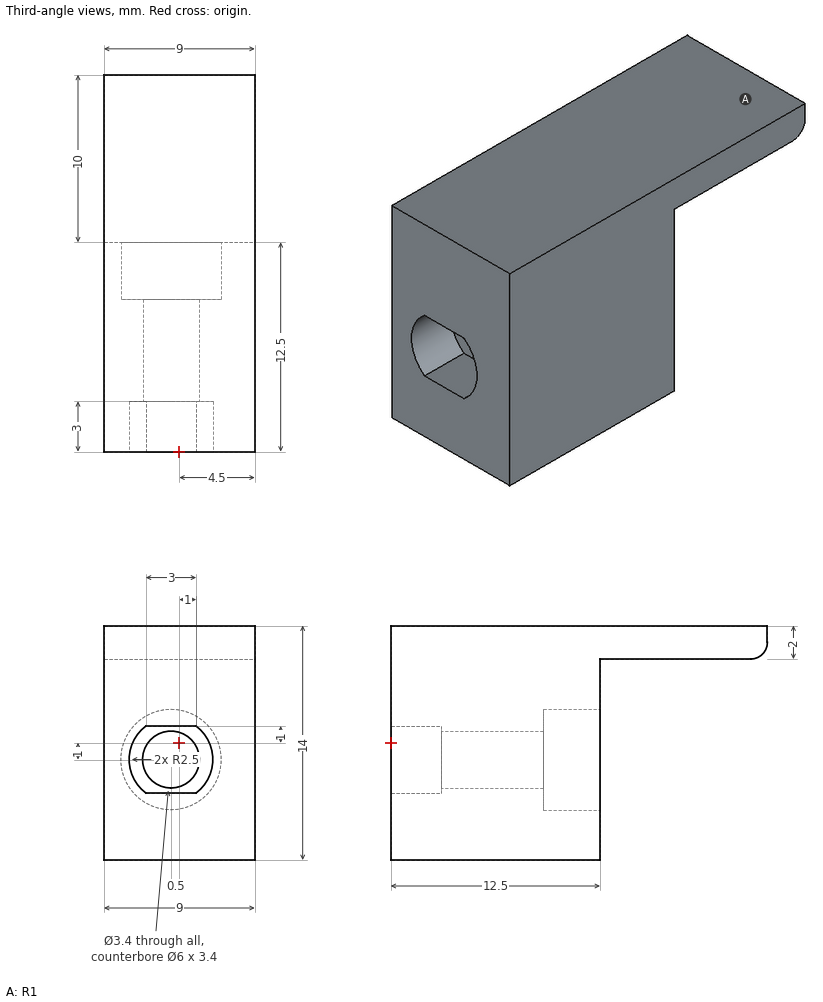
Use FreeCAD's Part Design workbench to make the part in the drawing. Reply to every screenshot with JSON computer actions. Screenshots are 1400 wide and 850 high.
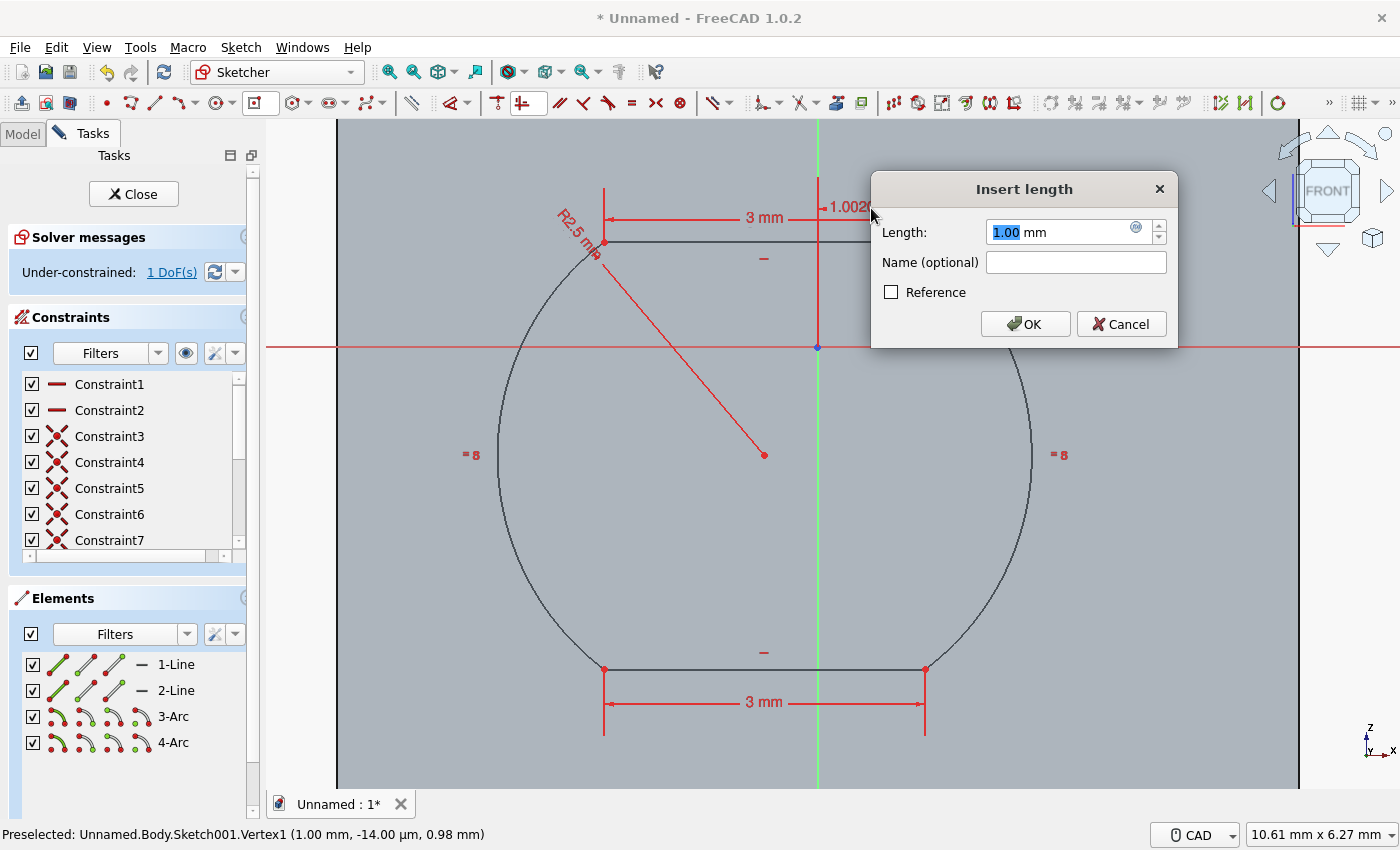
{"action": "type", "text": "1"}
{"action": "key", "text": "Return"}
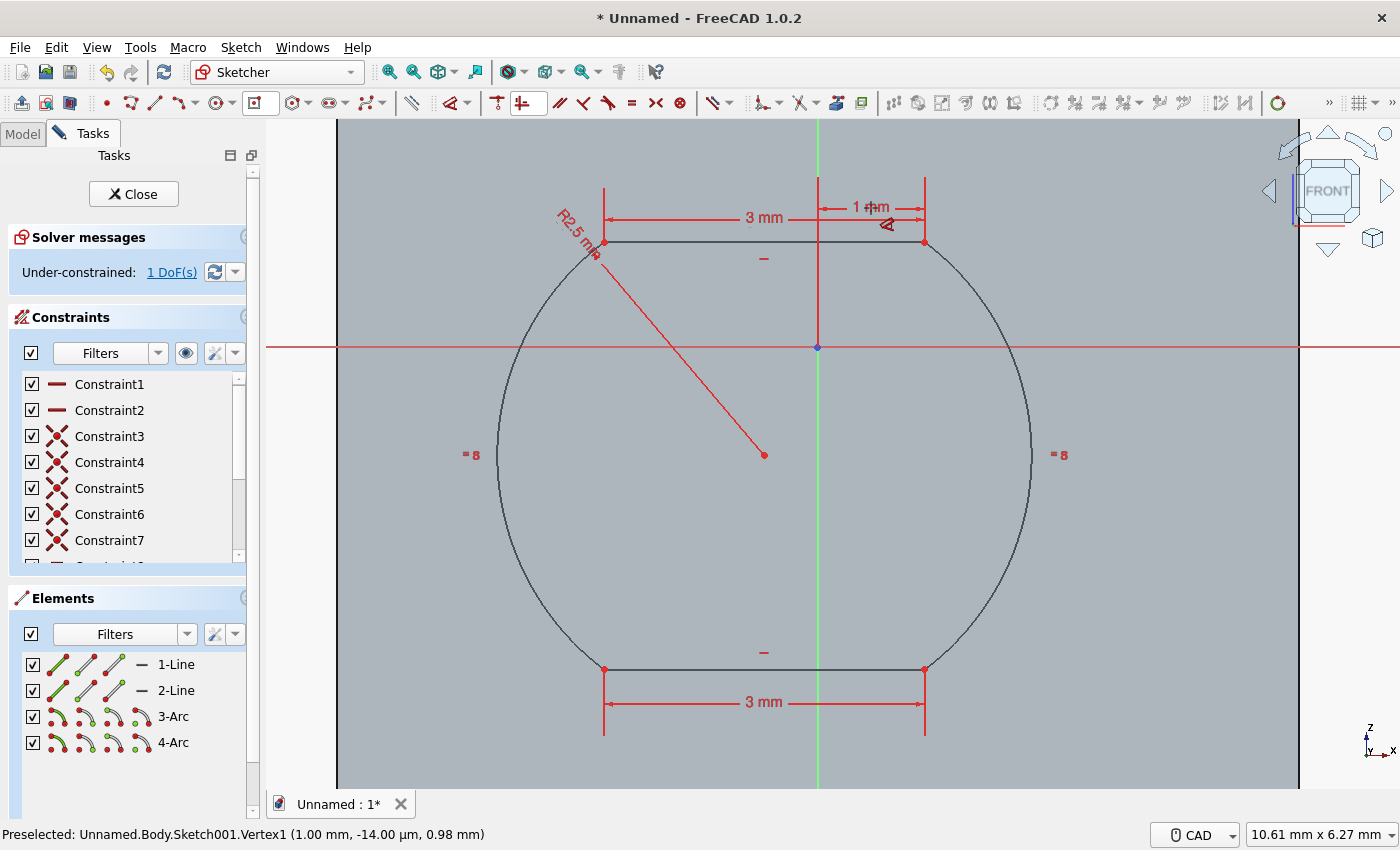
{"action": "left_click", "coordinate": [925, 242]}
{"action": "left_click", "coordinate": [959, 295]}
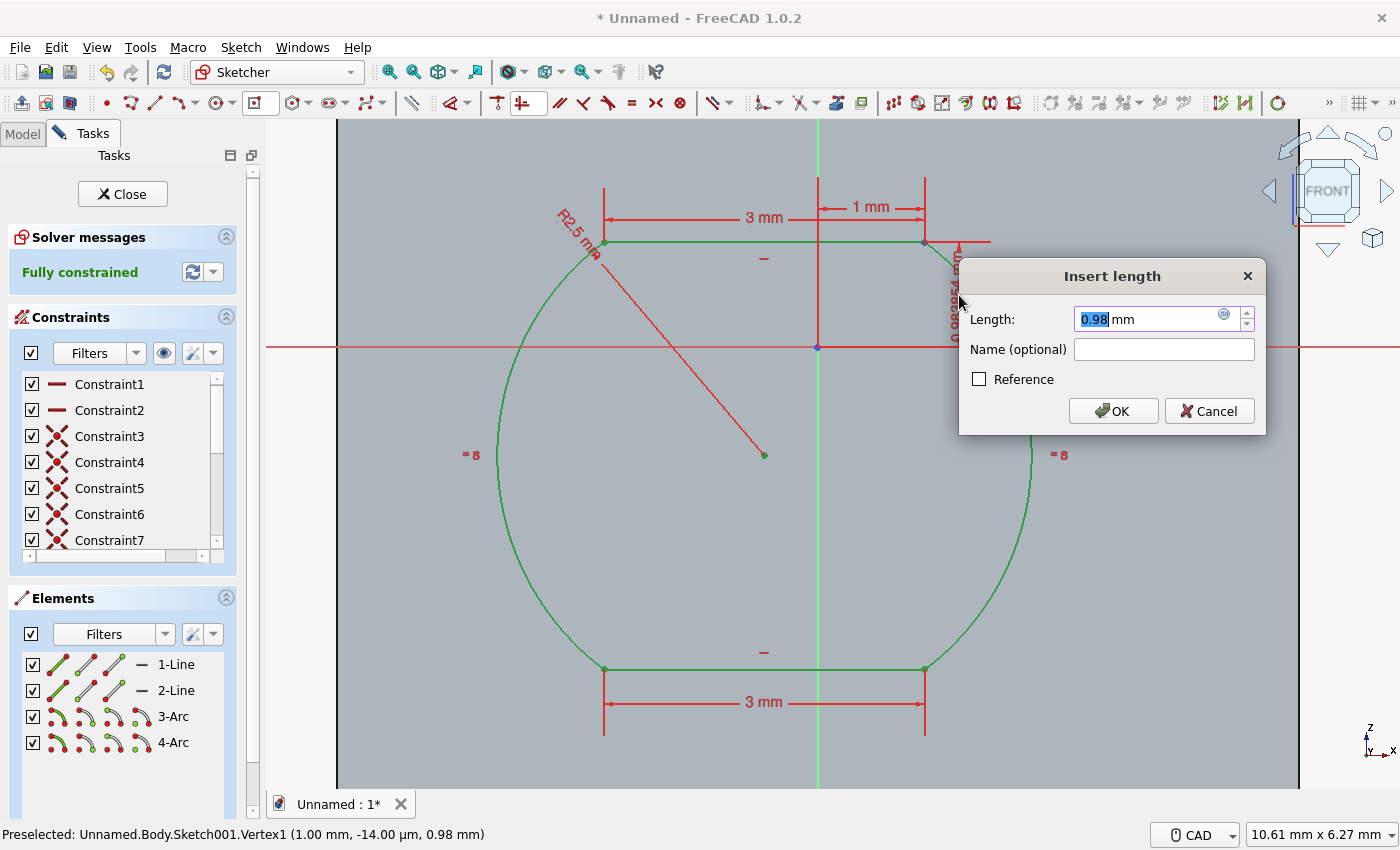
{"action": "type", "text": "1"}
{"action": "key", "text": "Return"}
{"action": "key", "text": "Escape"}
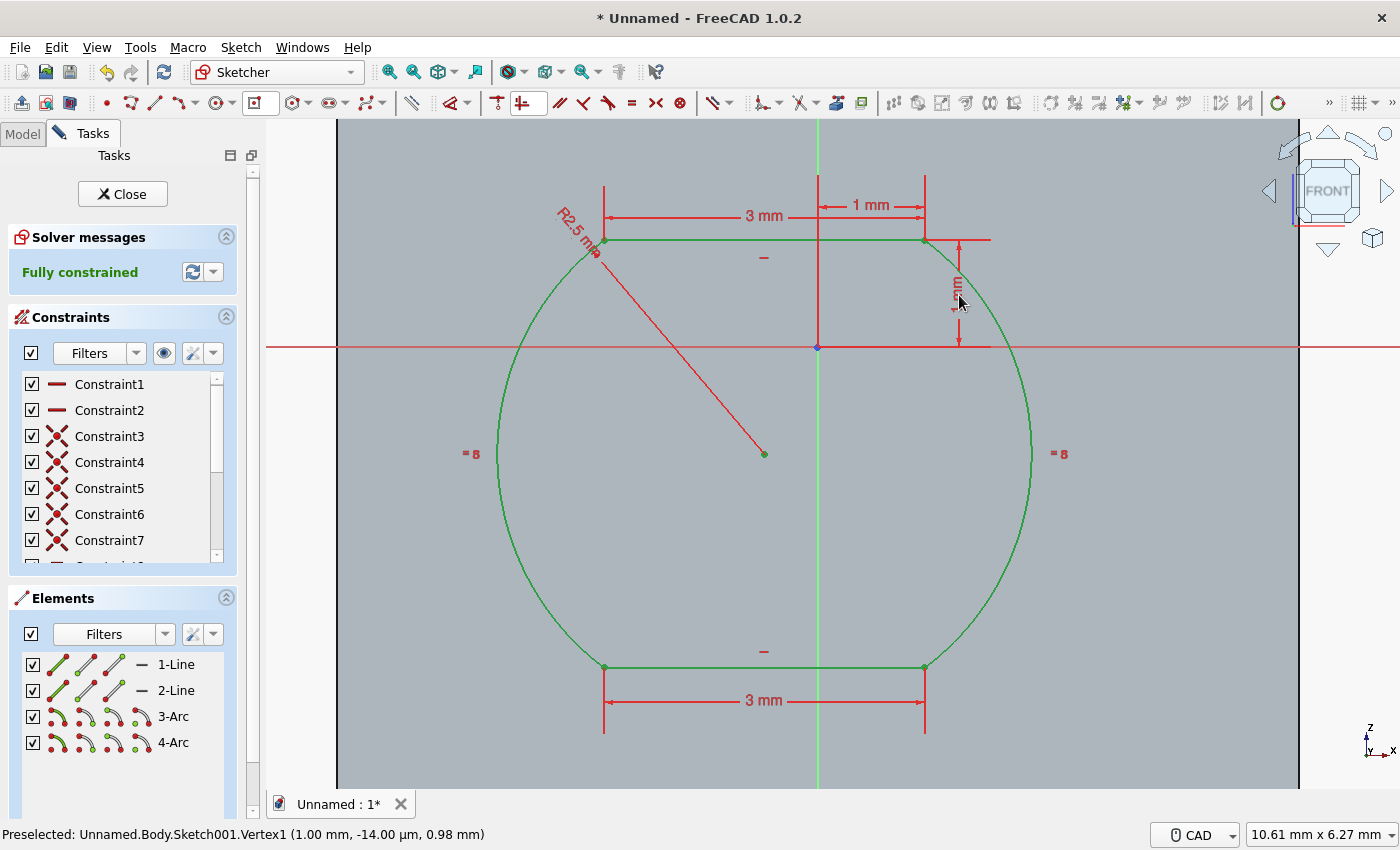
{"action": "left_click", "coordinate": [123, 194]}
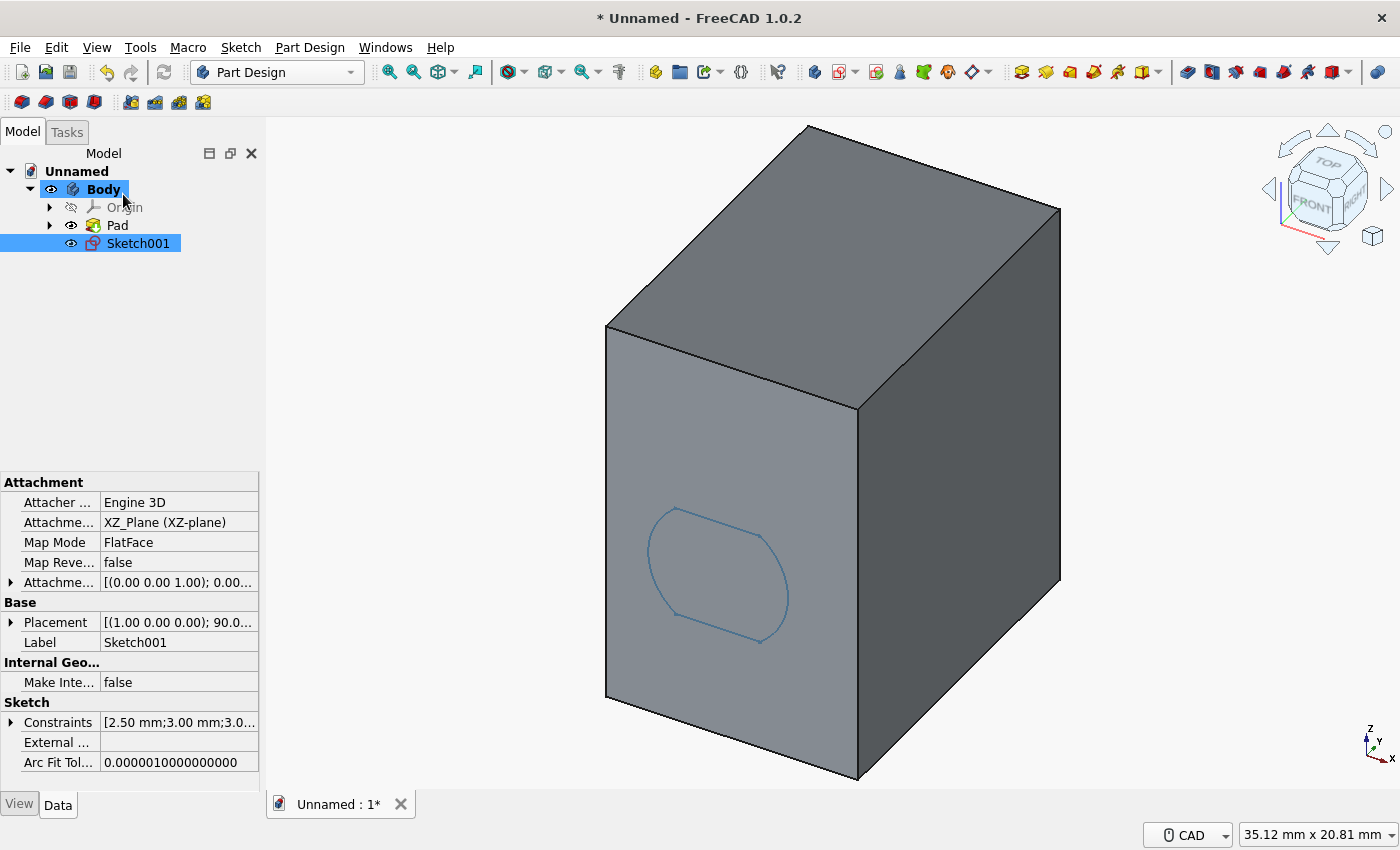
{"action": "left_click", "coordinate": [1188, 72]}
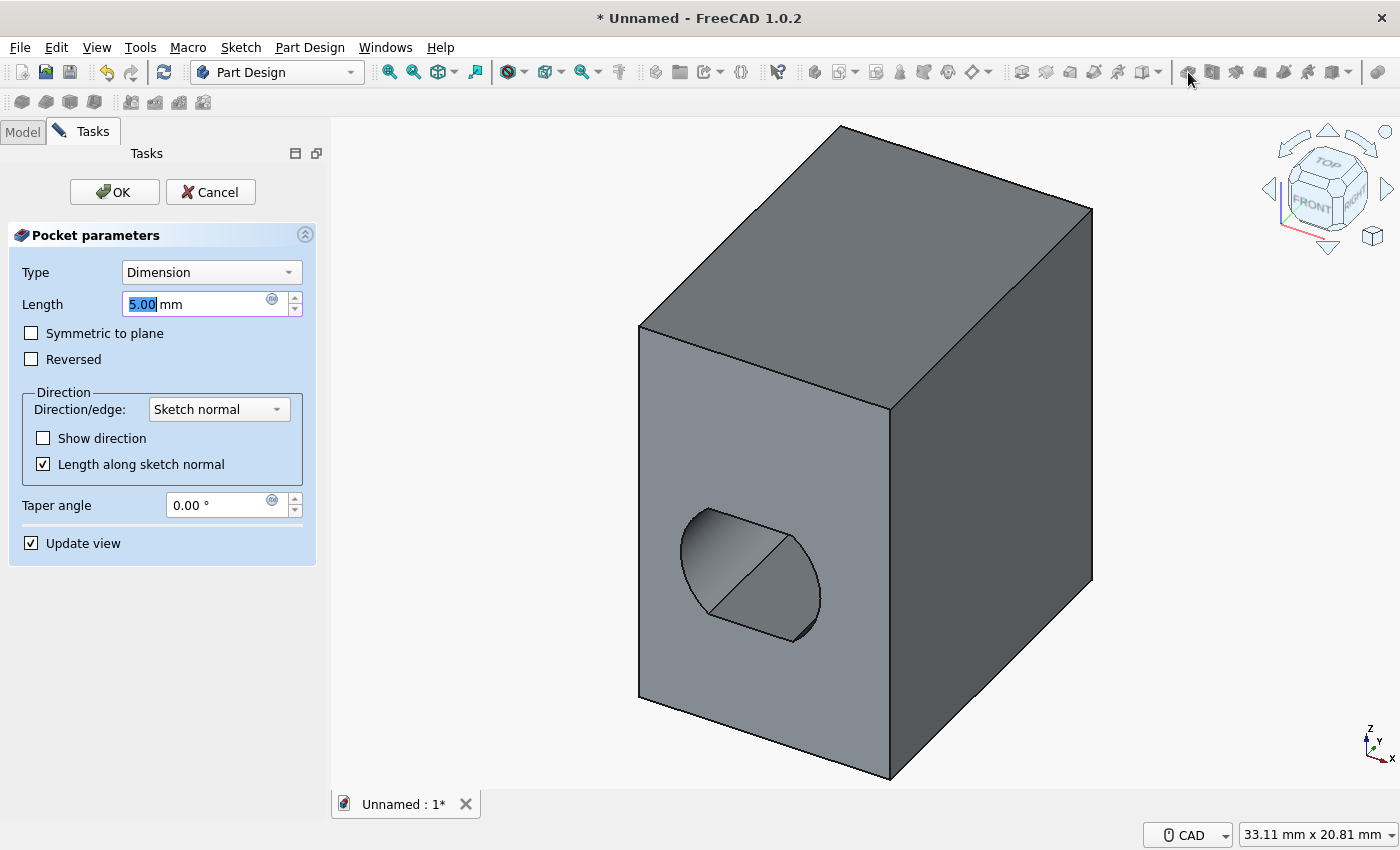
{"action": "type", "text": "3"}
{"action": "key", "text": "Tab"}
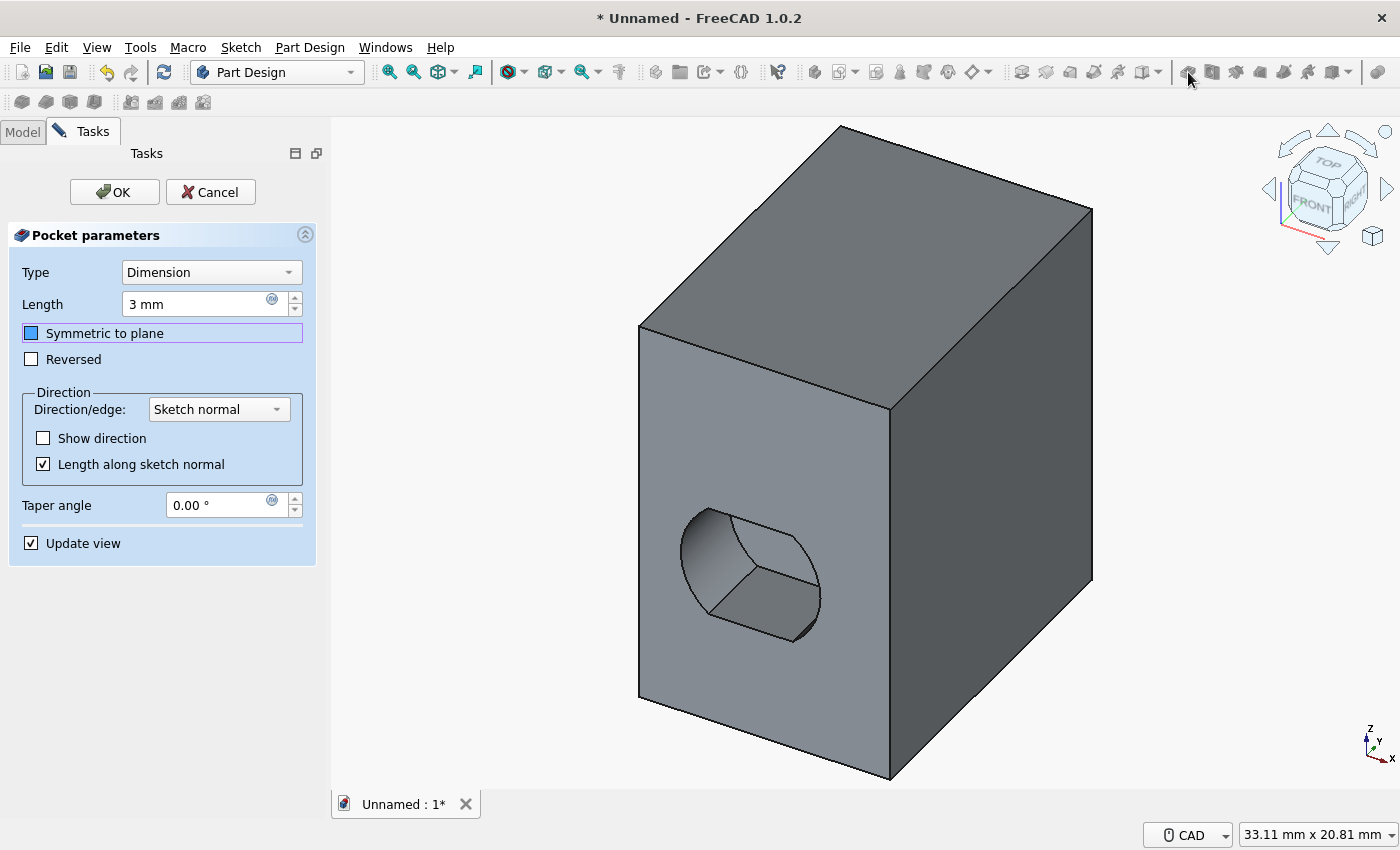
{"action": "left_click", "coordinate": [115, 192]}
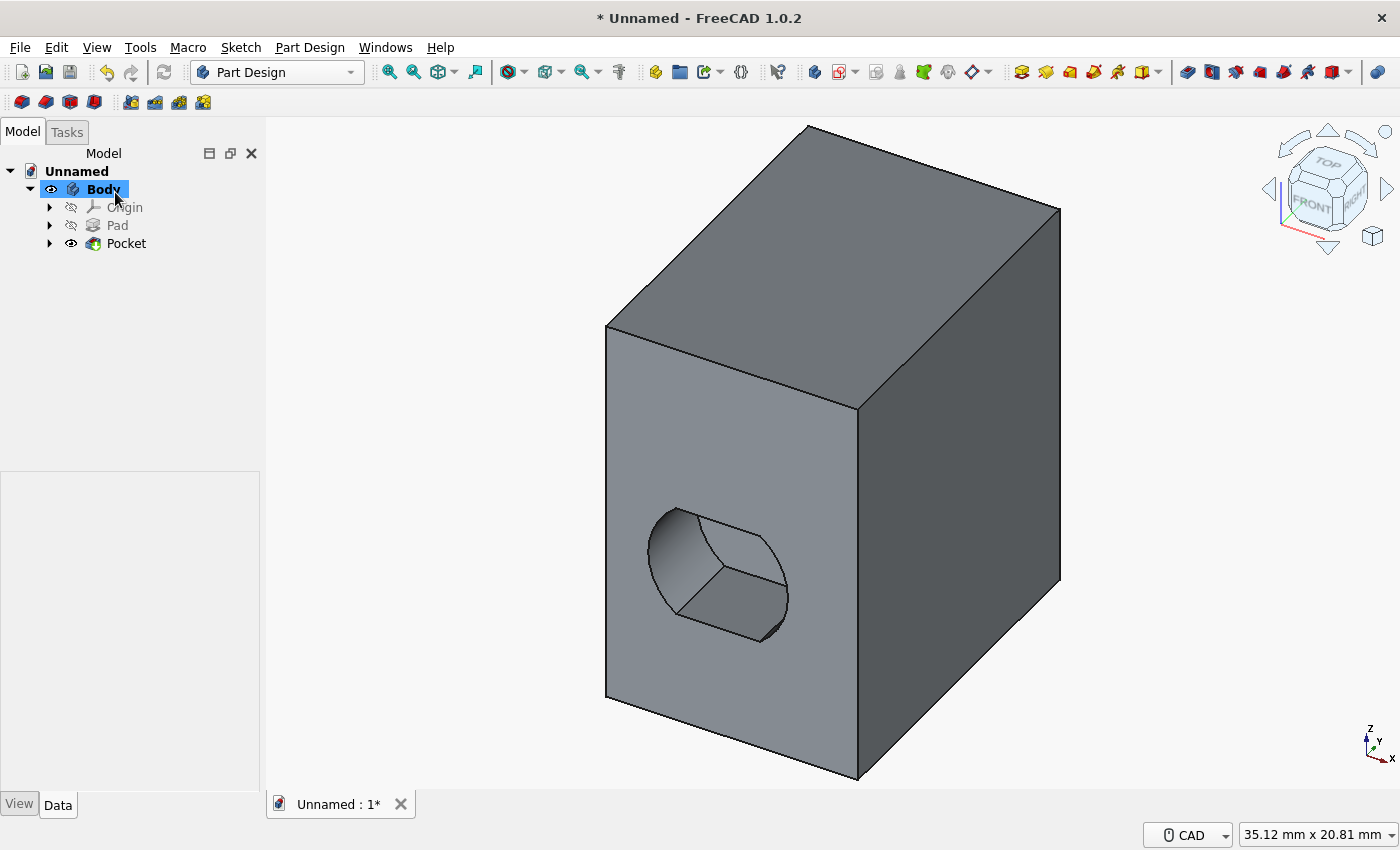
{"action": "left_click", "coordinate": [833, 267]}